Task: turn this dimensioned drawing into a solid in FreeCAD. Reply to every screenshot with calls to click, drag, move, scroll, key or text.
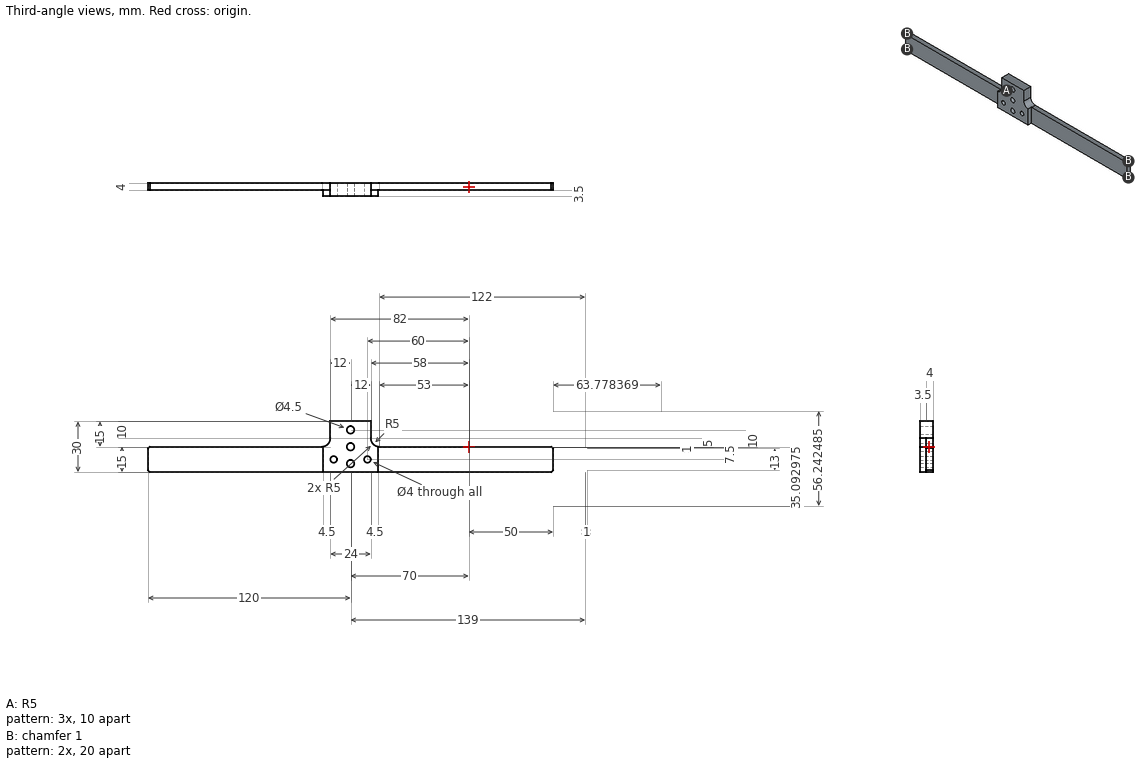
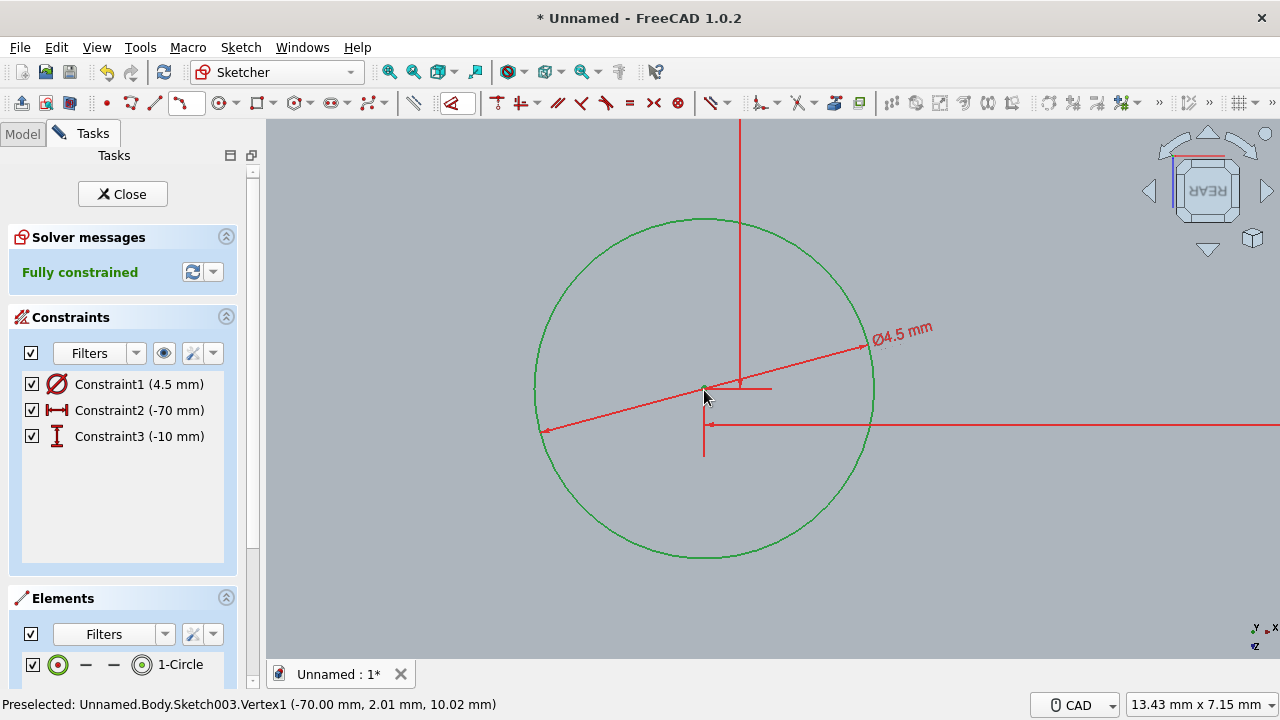
click(123, 194)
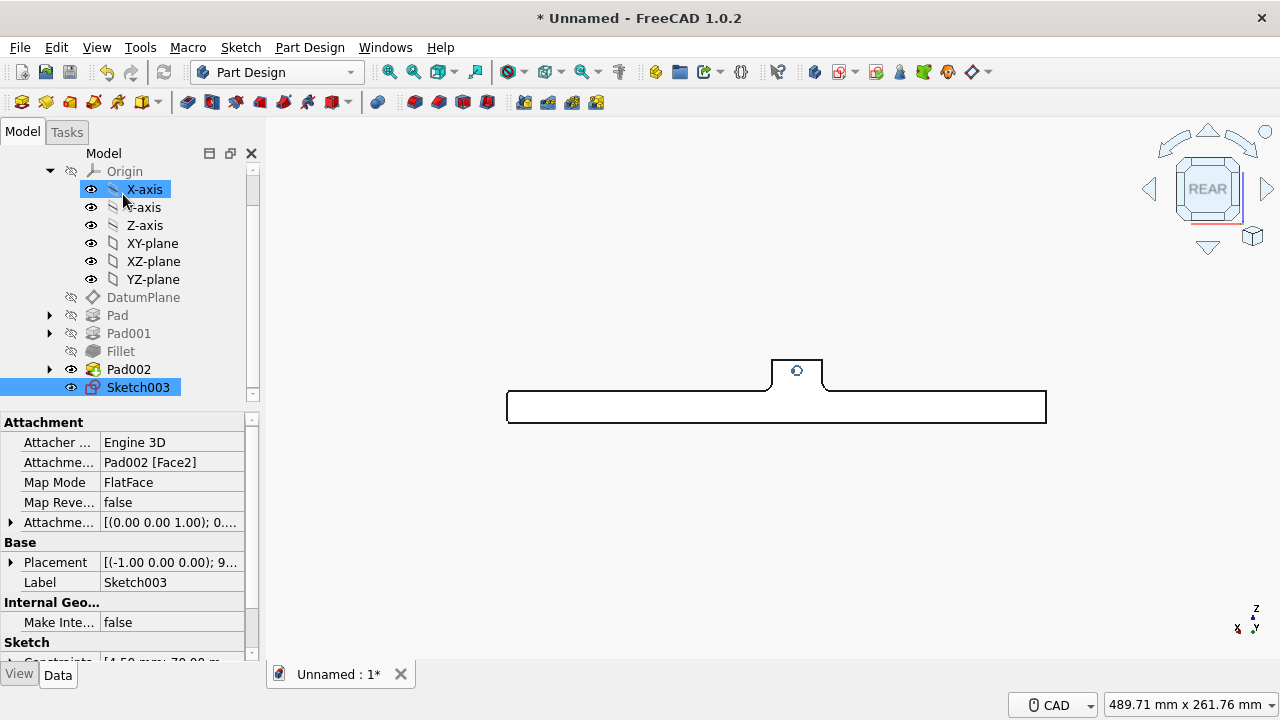
click(188, 102)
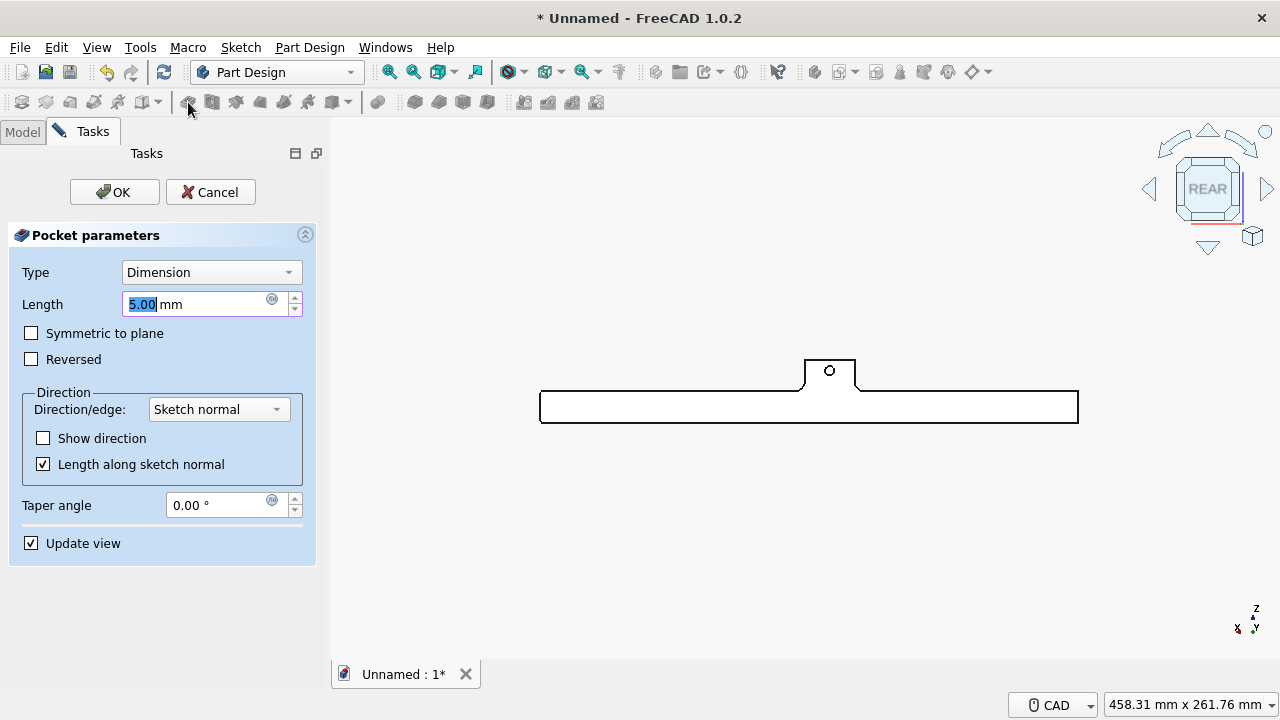
click(212, 272)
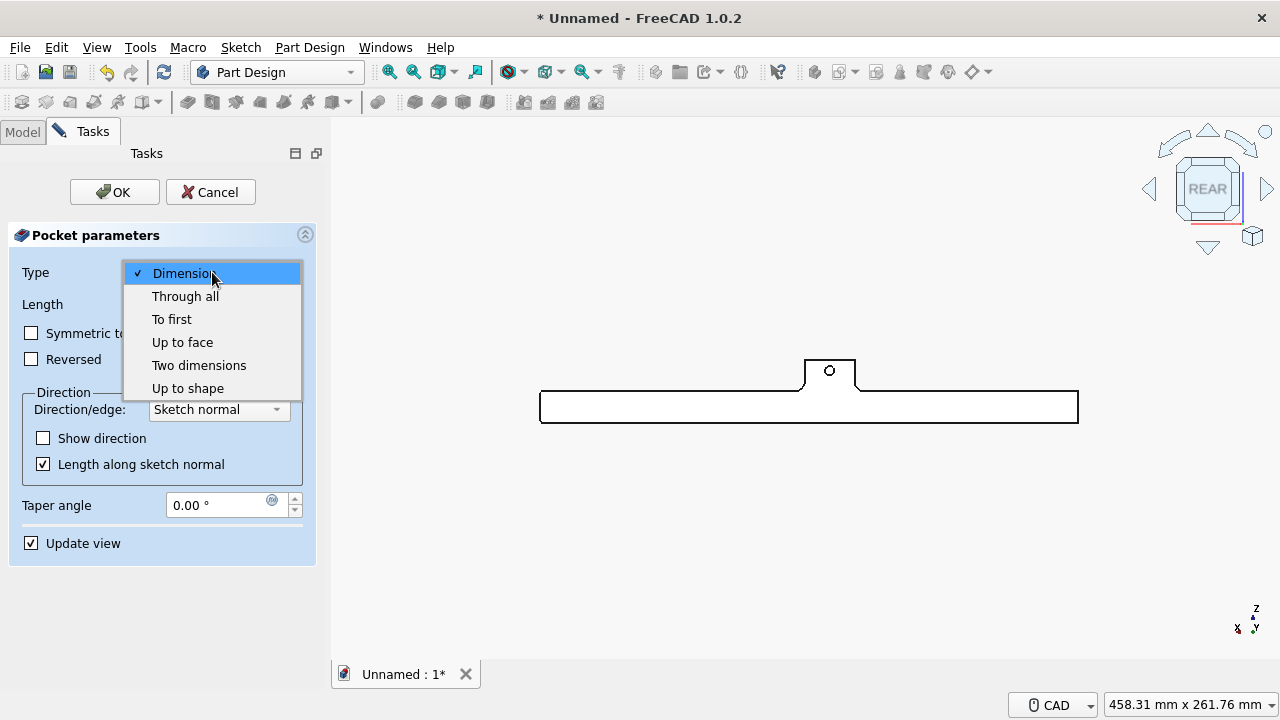
click(212, 296)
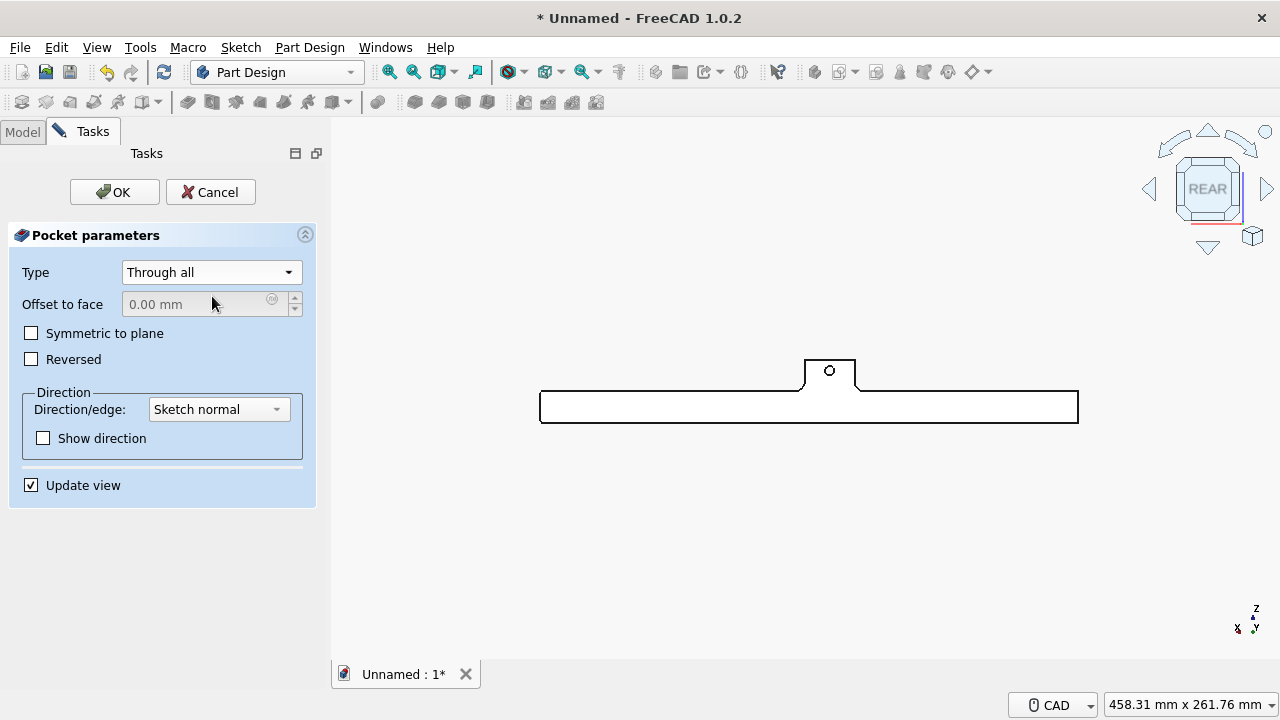
click(115, 192)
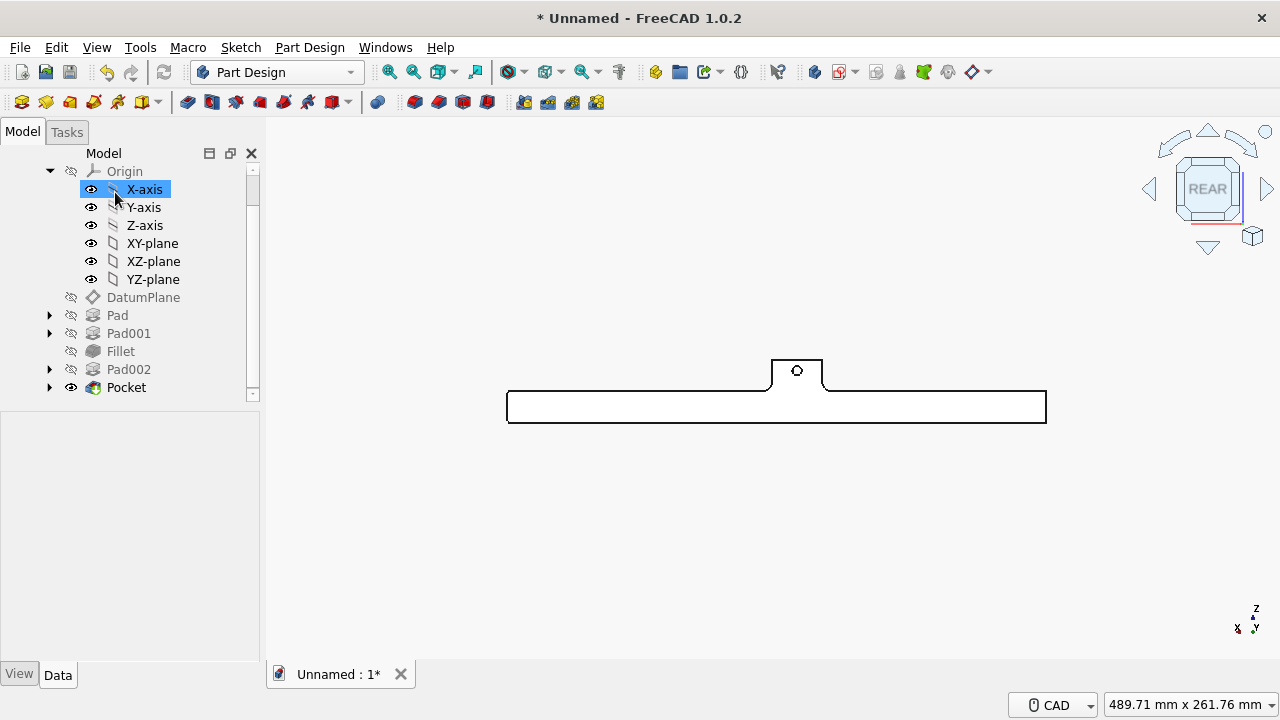
click(116, 387)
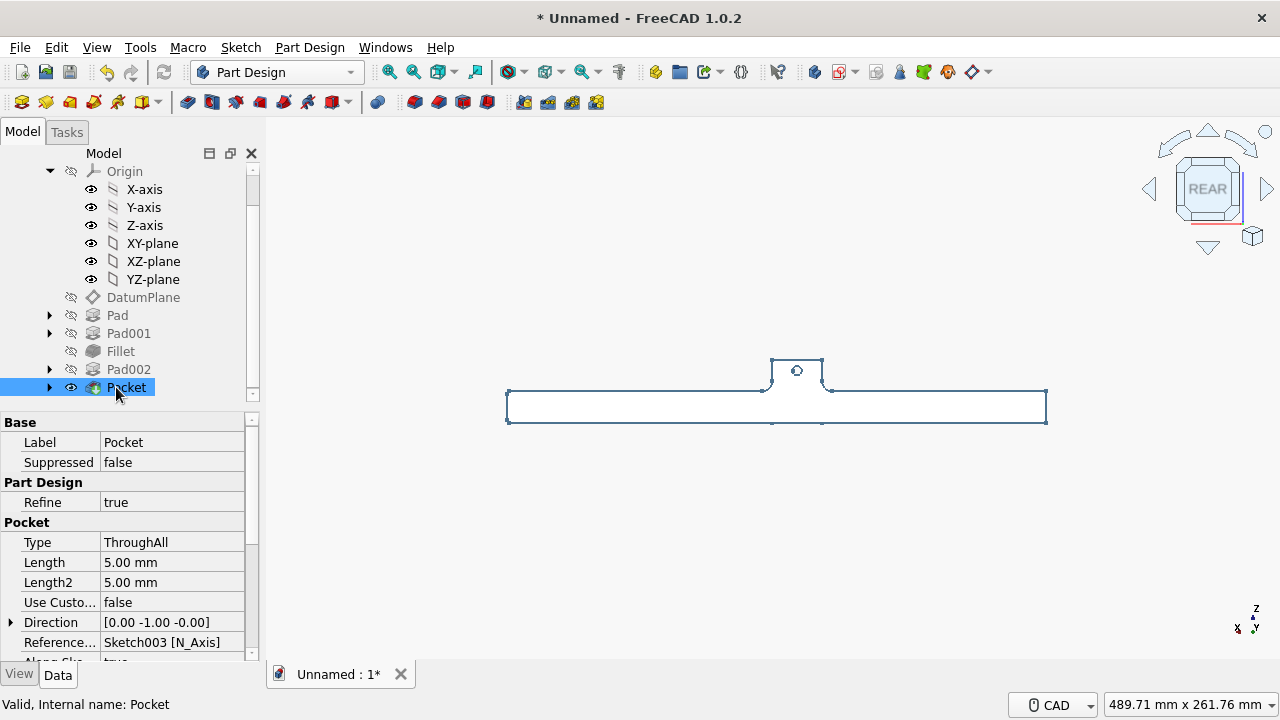
click(548, 102)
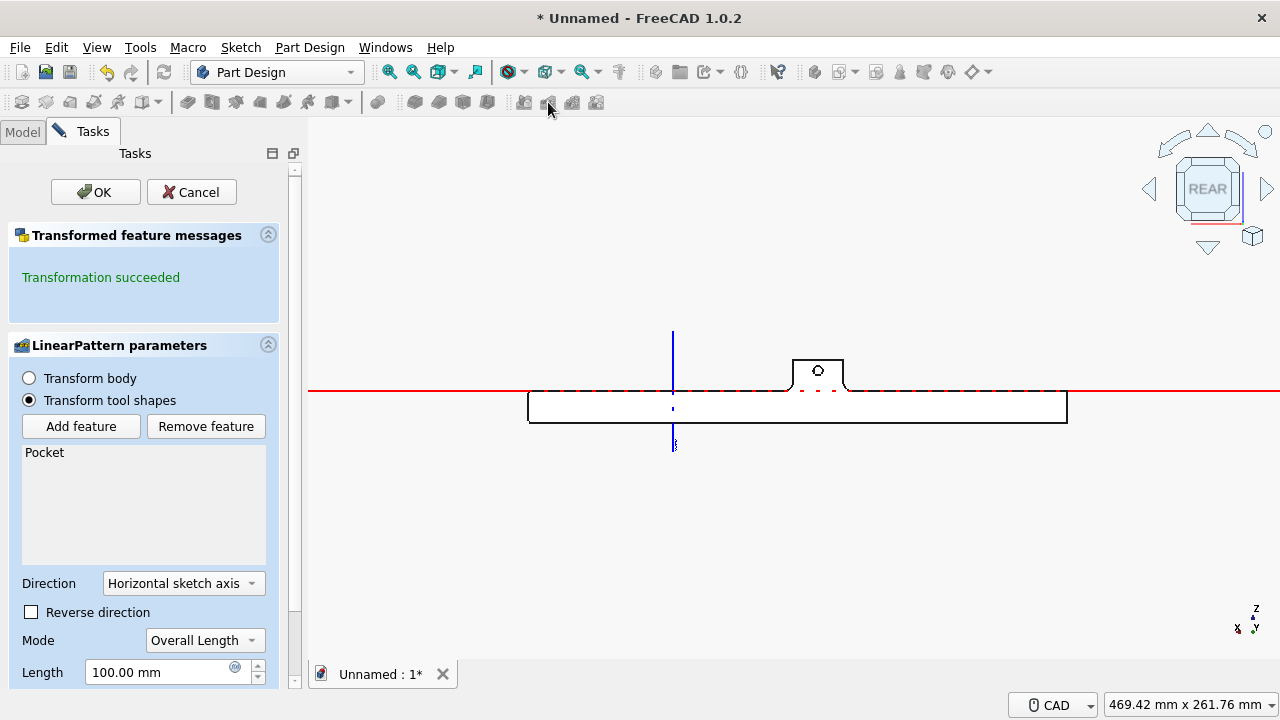
click(184, 584)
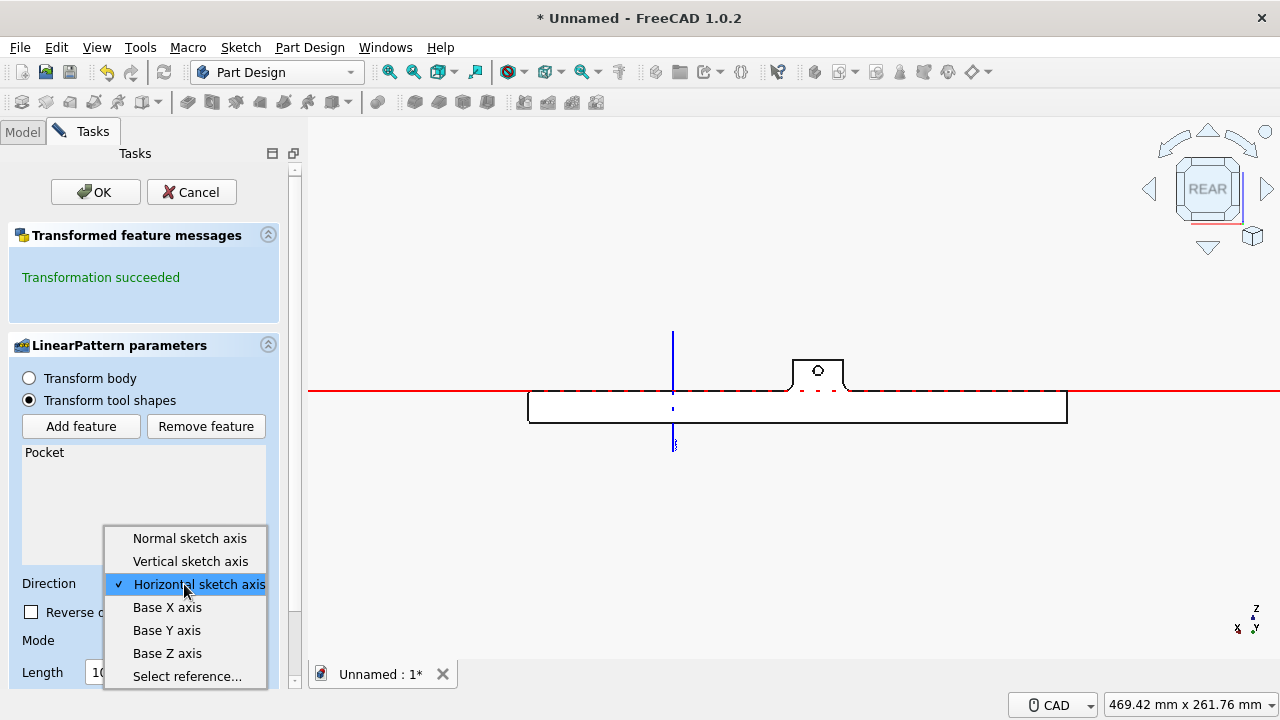
click(184, 654)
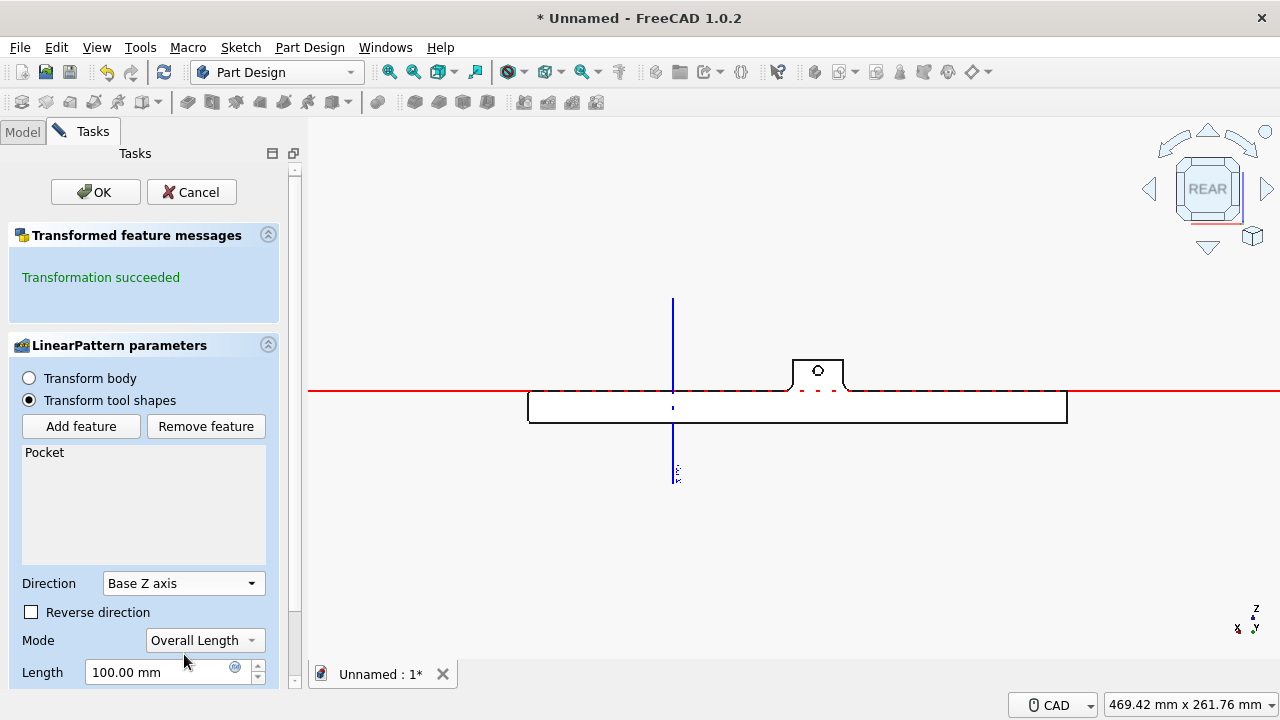
click(206, 640)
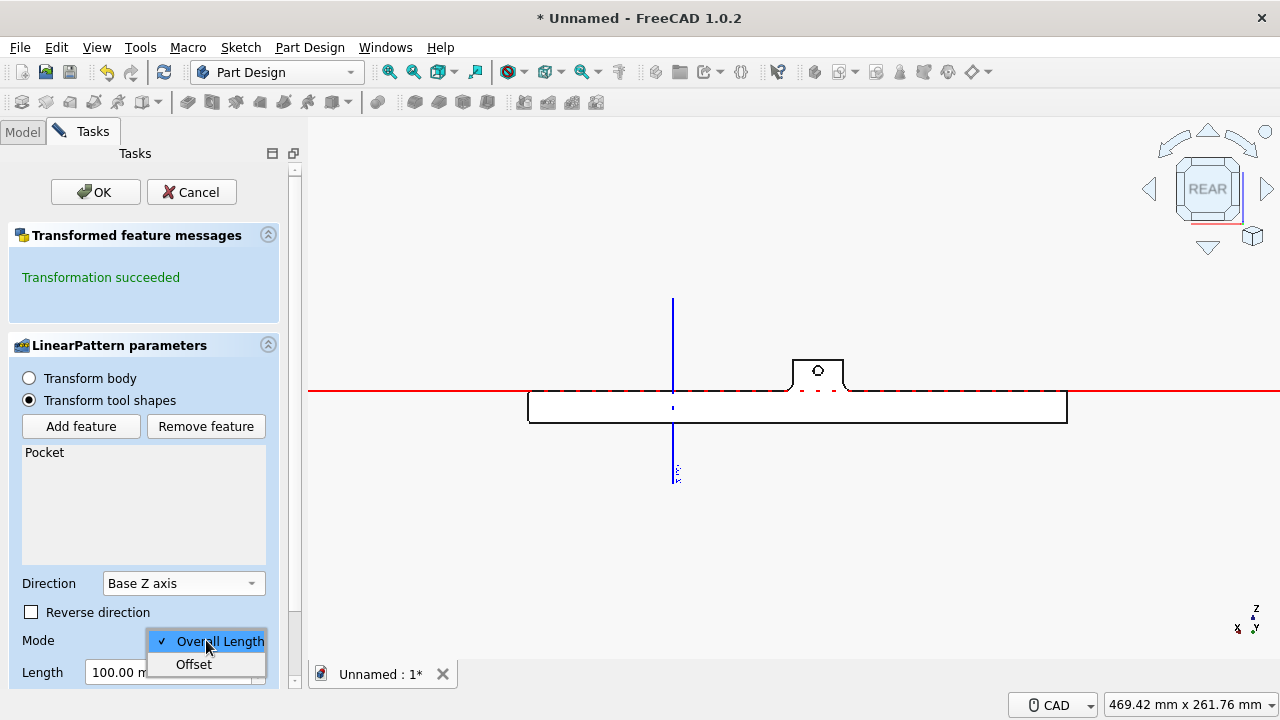
click(206, 664)